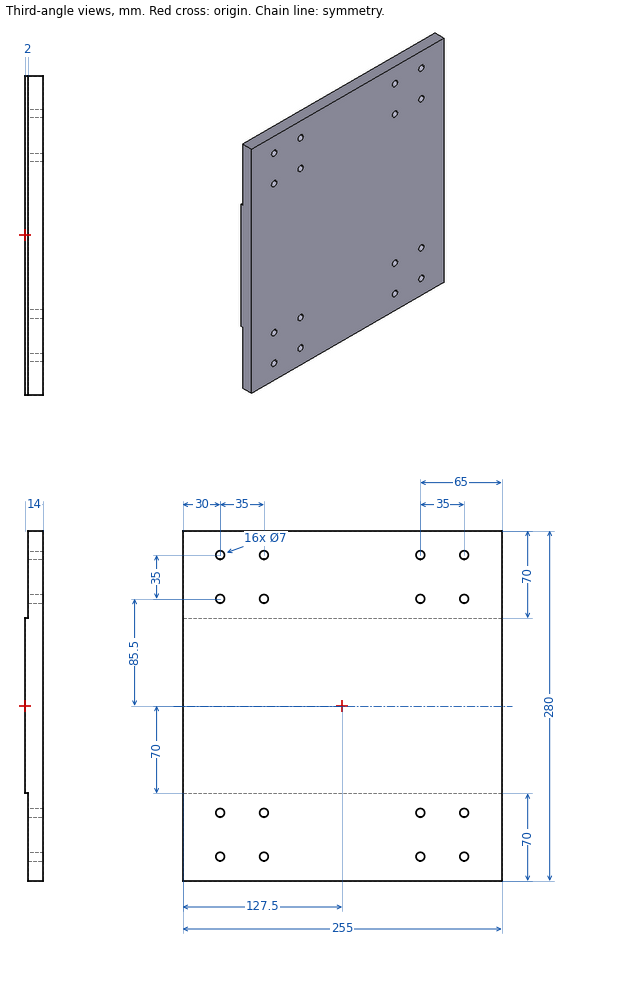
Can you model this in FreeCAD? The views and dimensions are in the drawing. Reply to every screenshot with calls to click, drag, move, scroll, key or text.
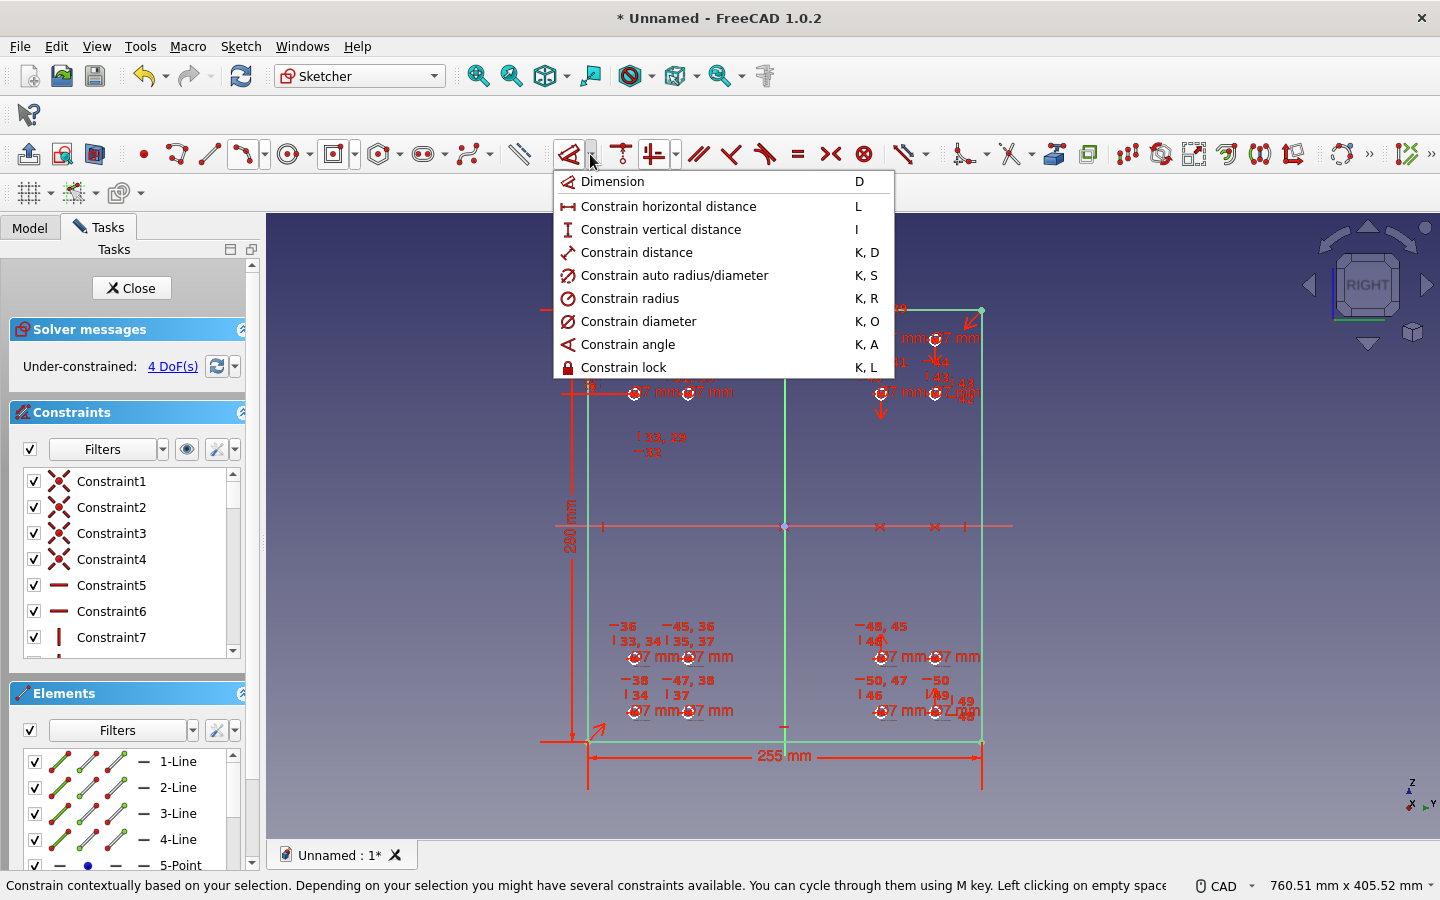
click(724, 206)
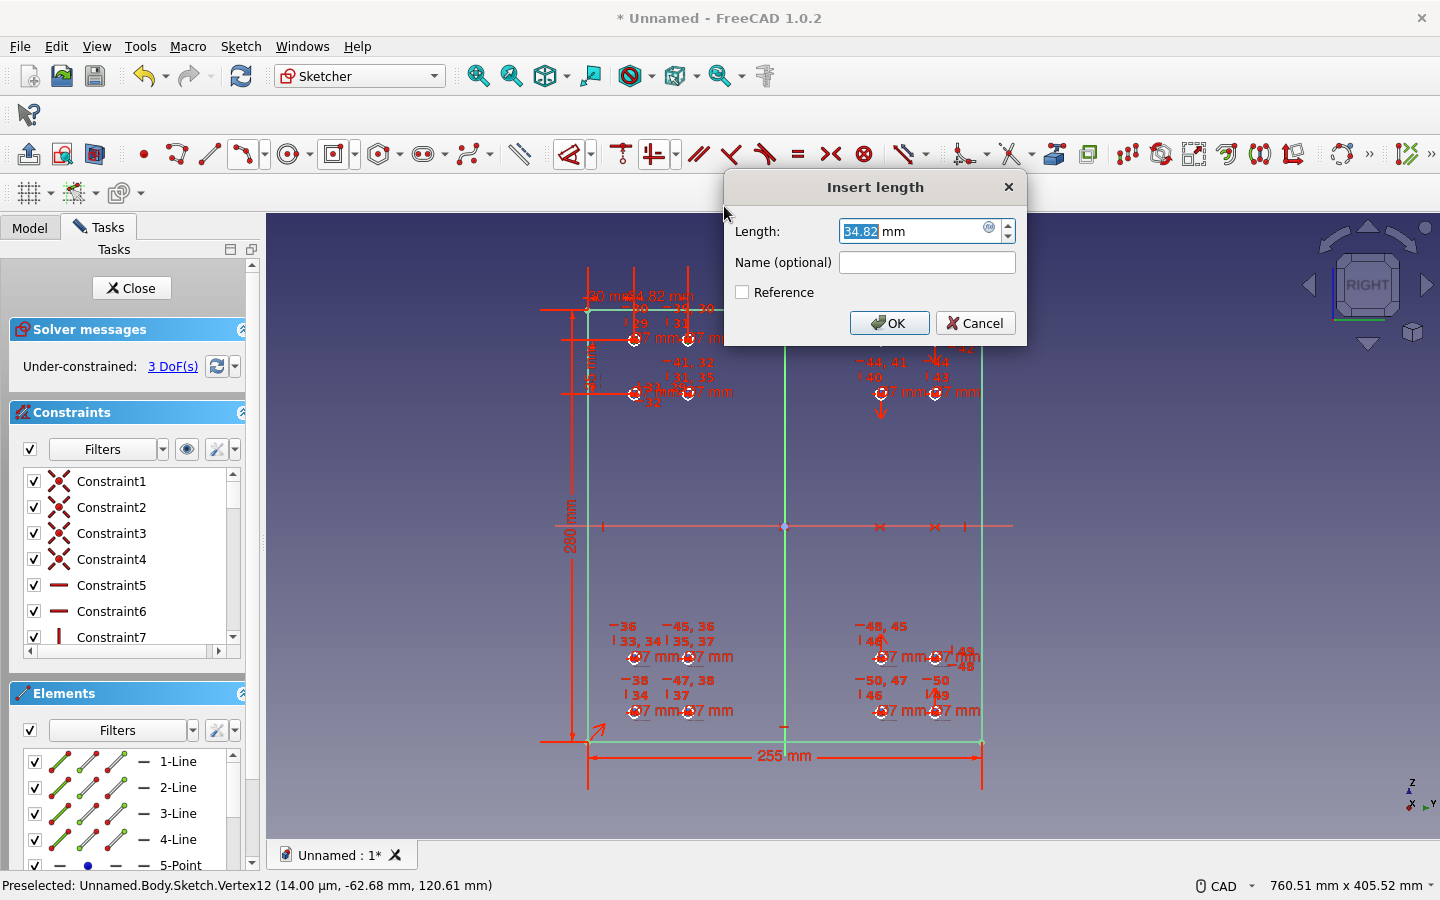
text(35)
key(Return)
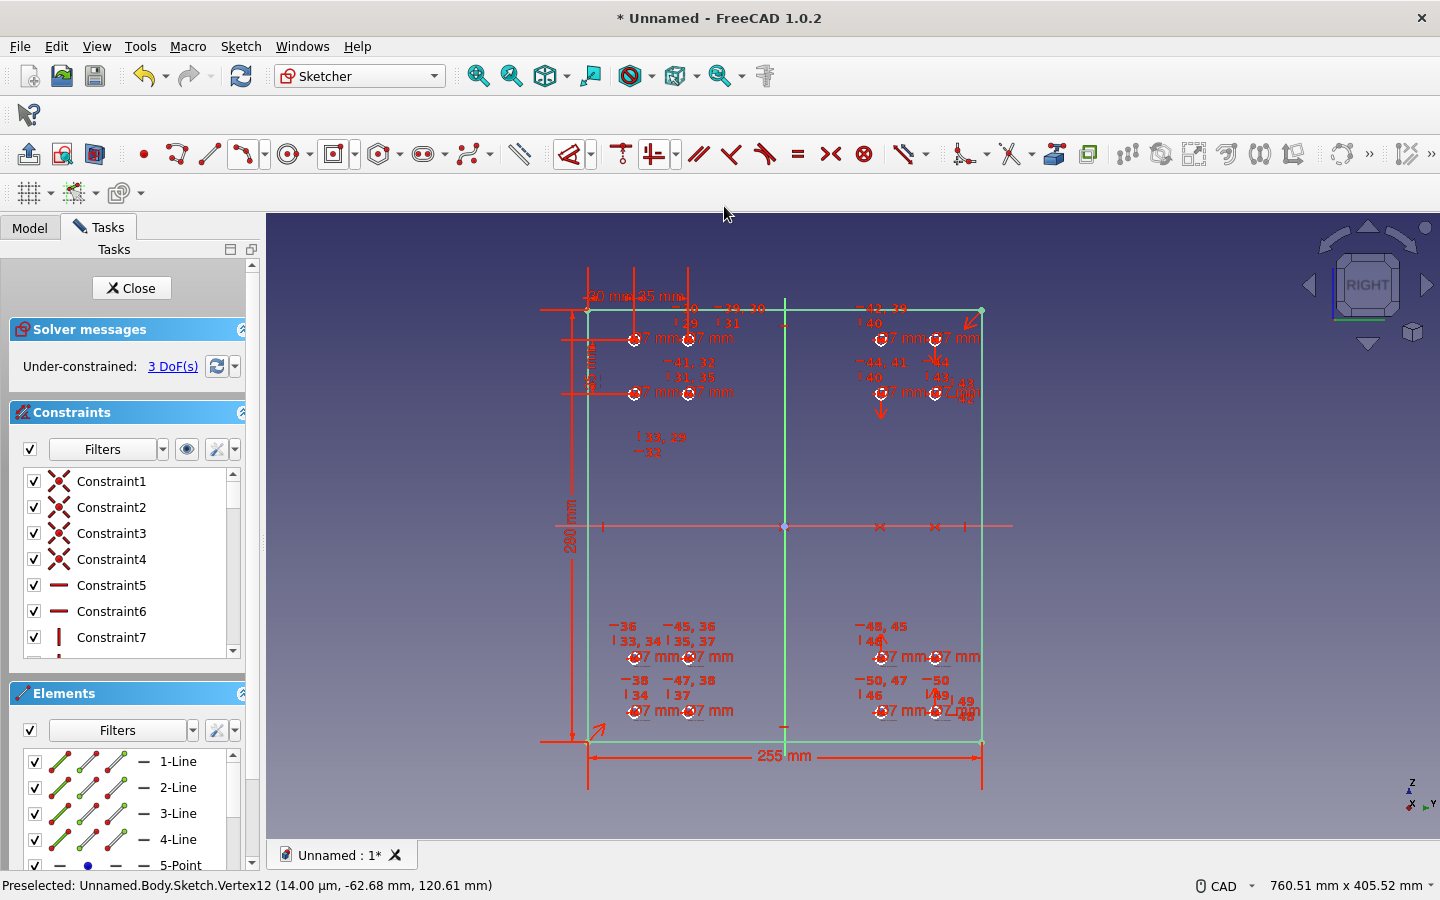
click(982, 310)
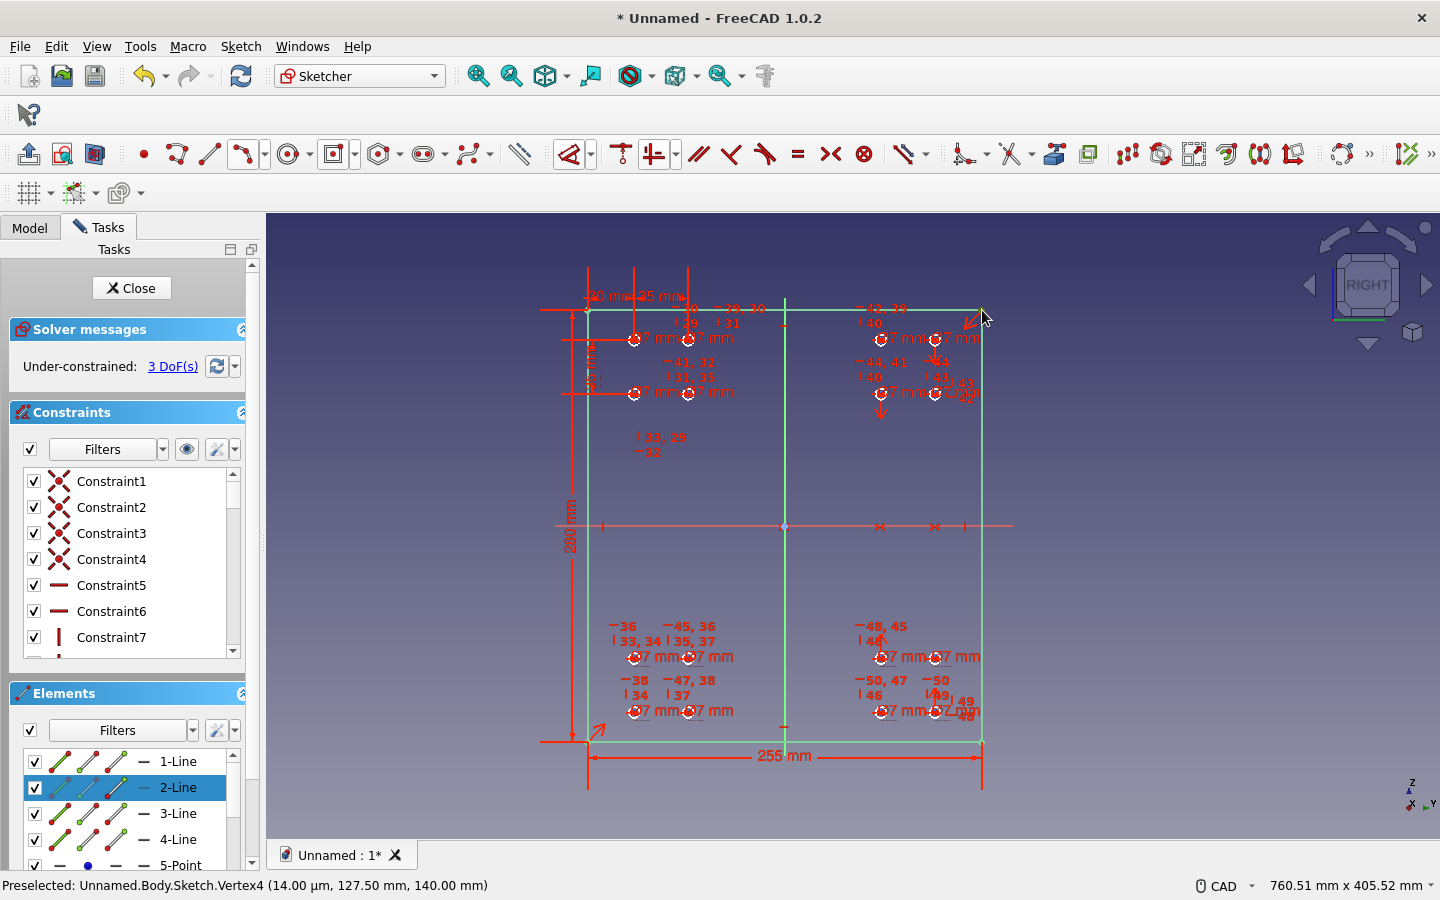
click(881, 340)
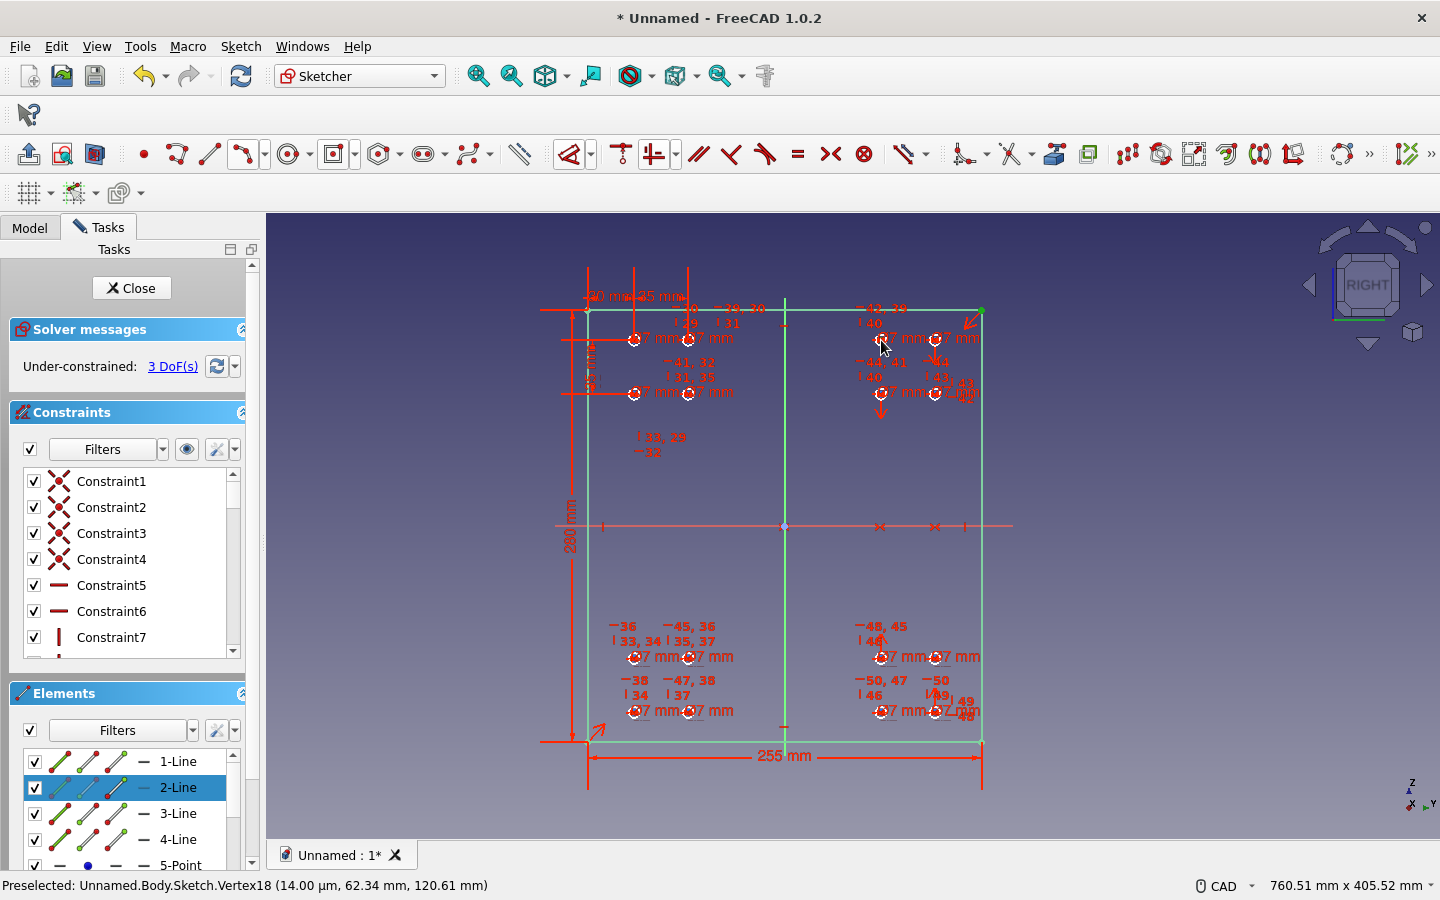
click(590, 154)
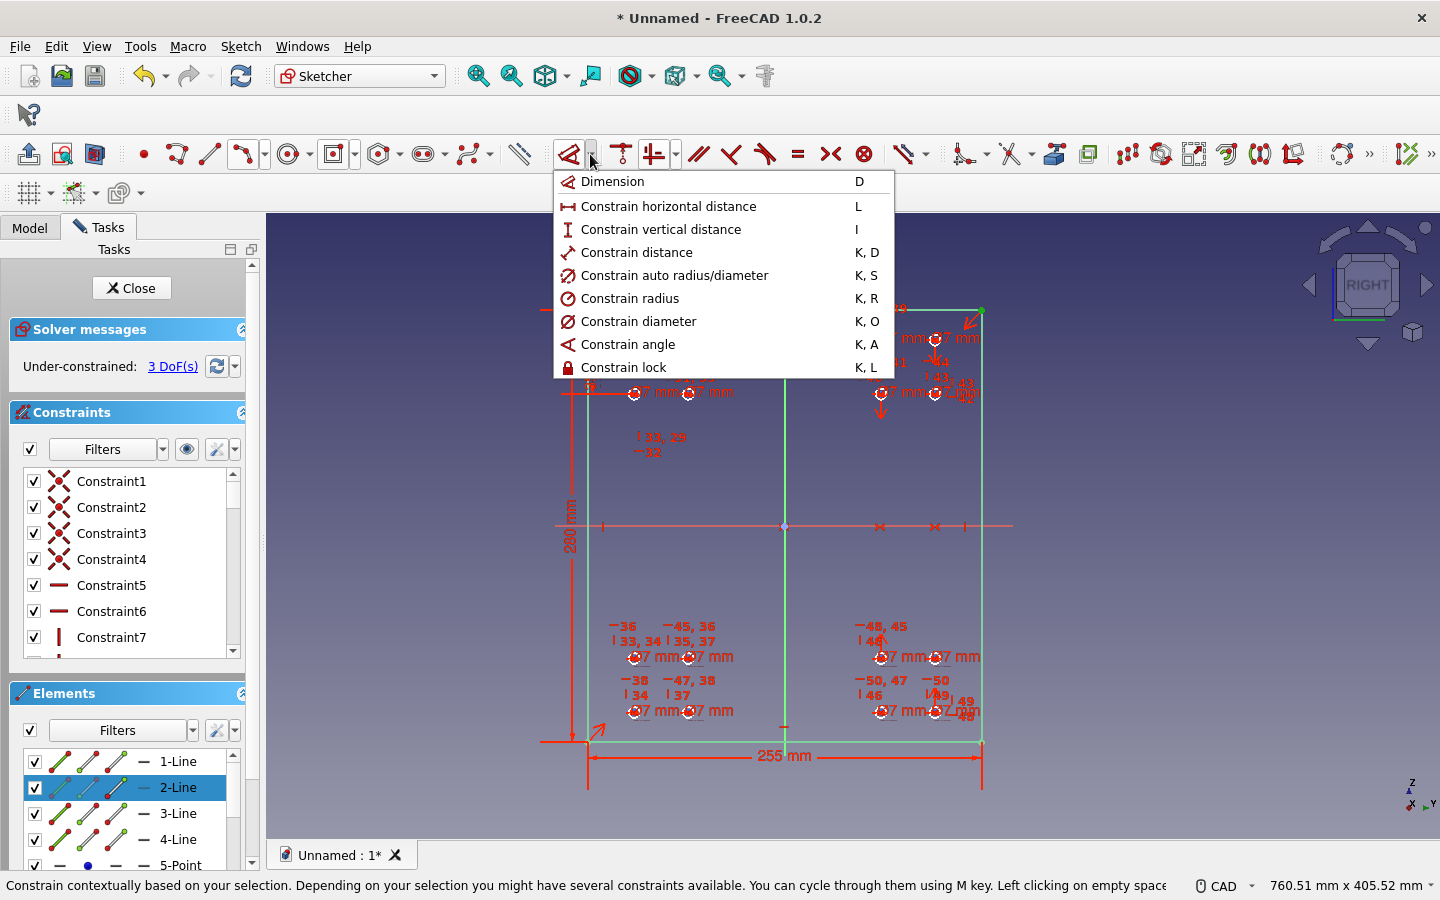
click(724, 206)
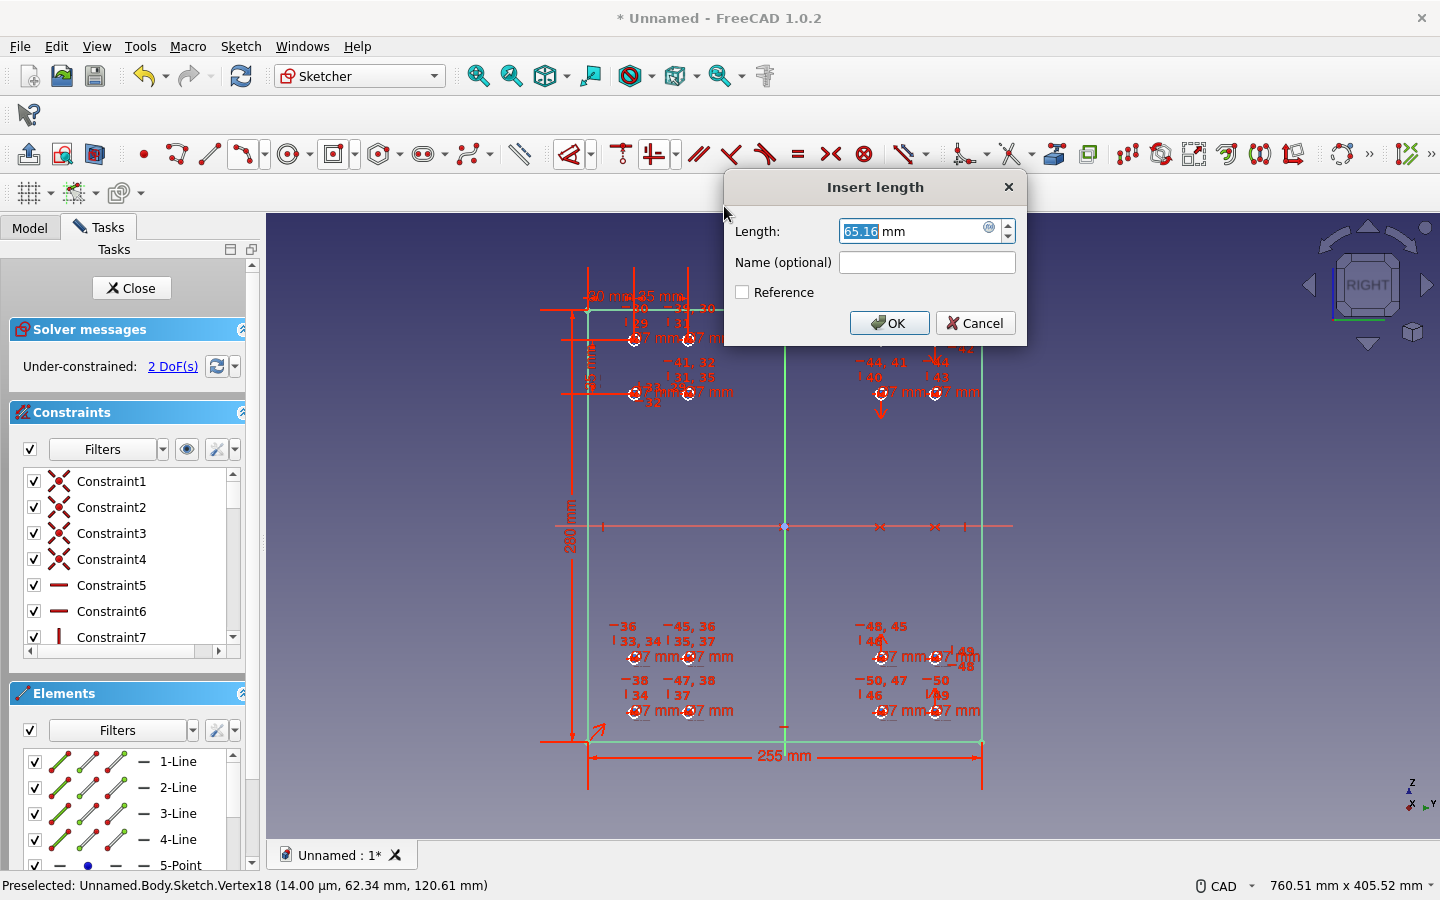
text(65)
key(Return)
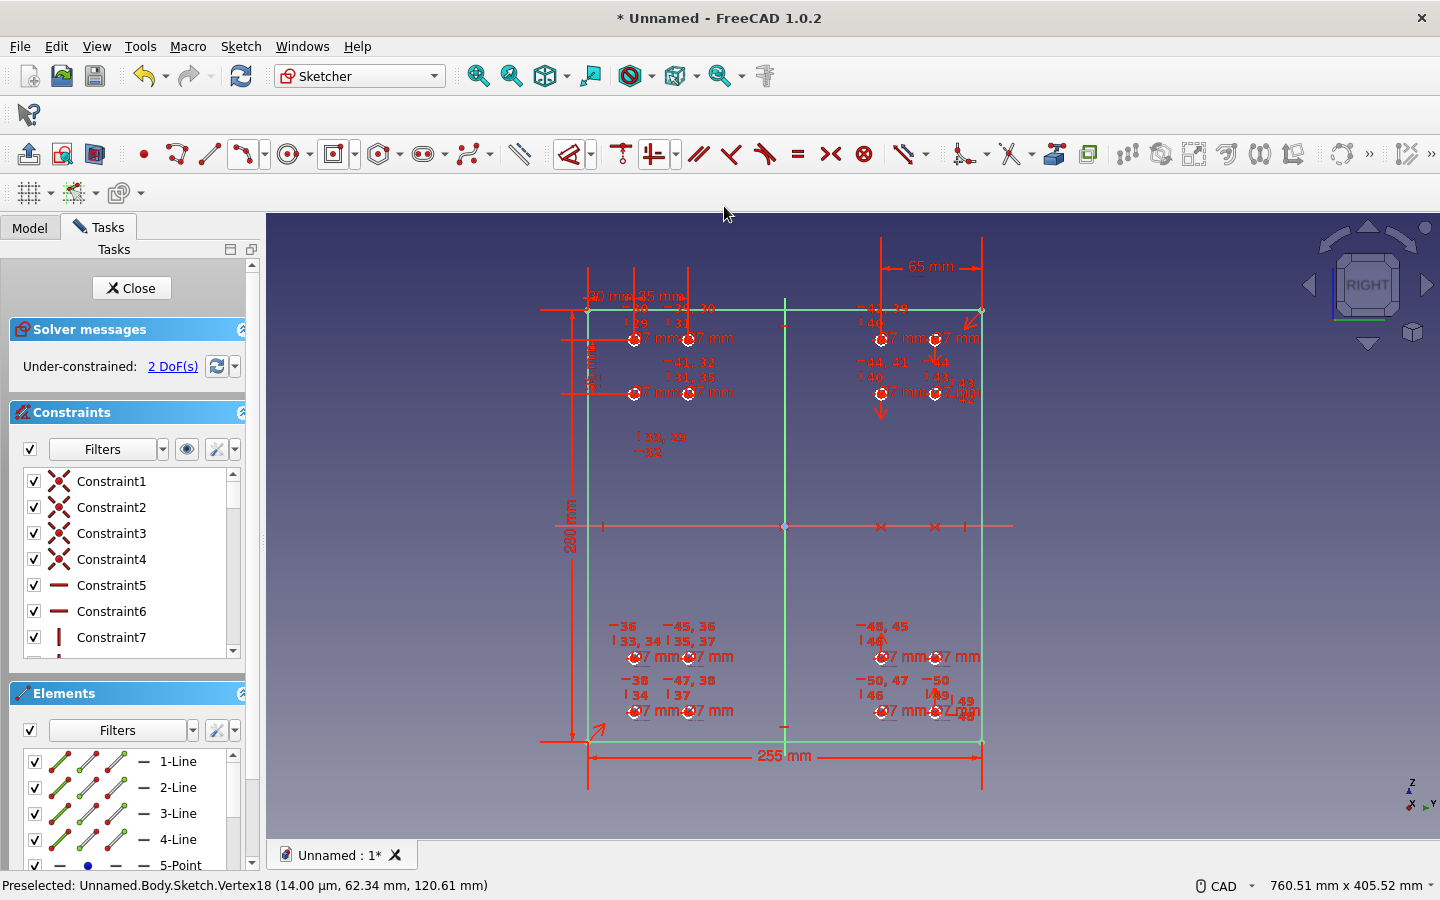
click(881, 340)